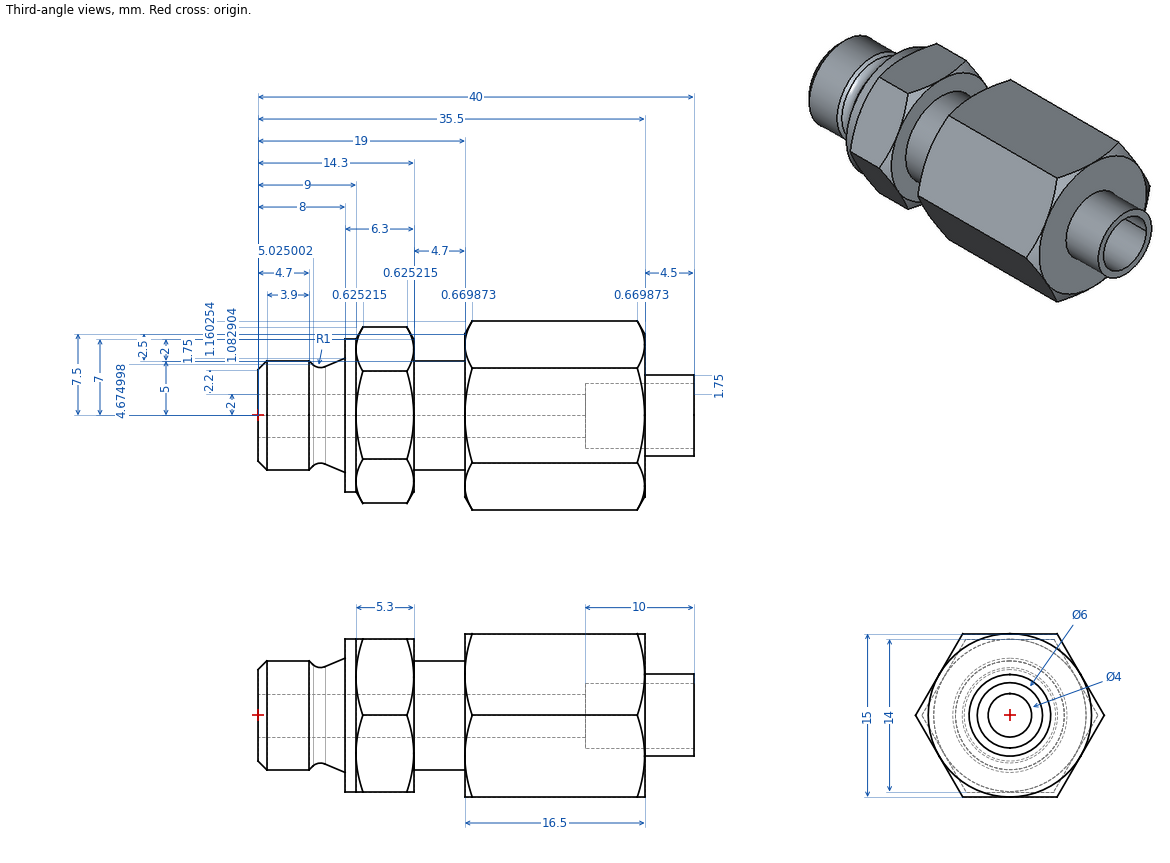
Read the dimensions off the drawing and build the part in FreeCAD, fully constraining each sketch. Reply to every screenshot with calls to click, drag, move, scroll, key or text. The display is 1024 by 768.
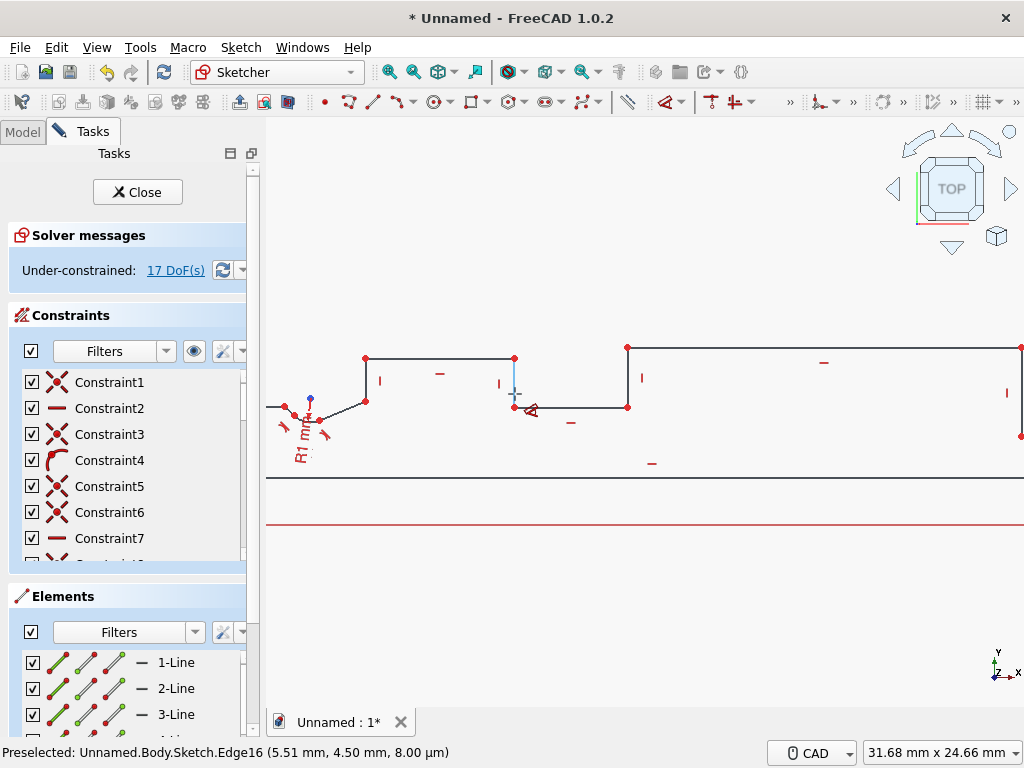
click(514, 393)
click(480, 383)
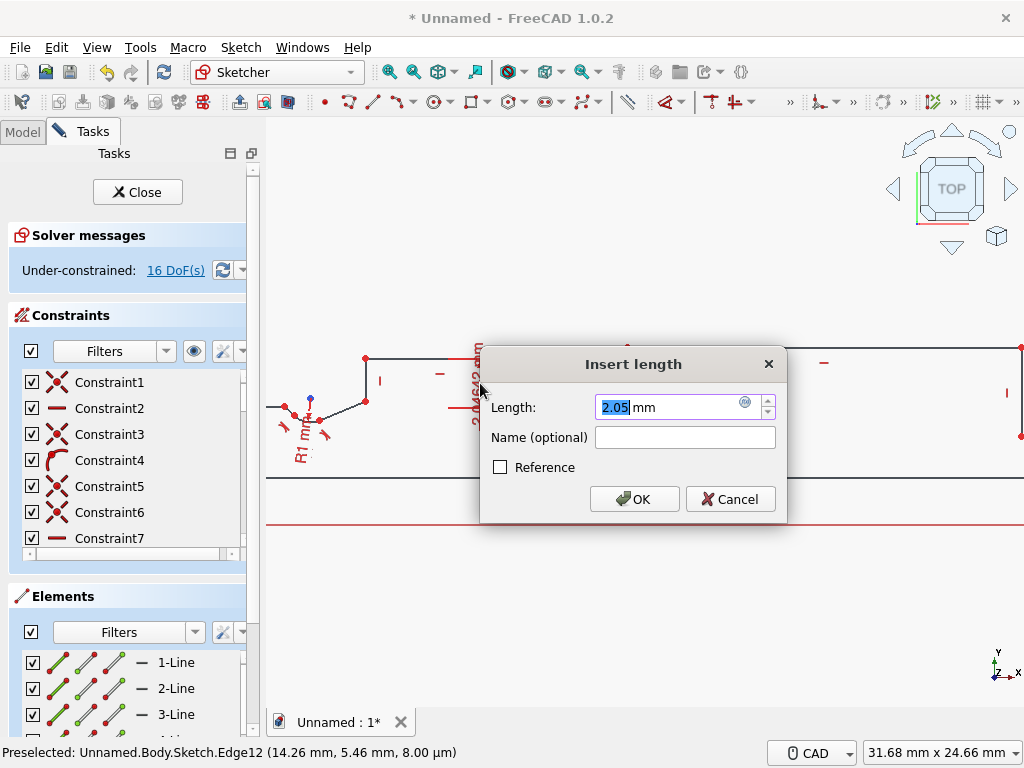
text(2)
key(Return)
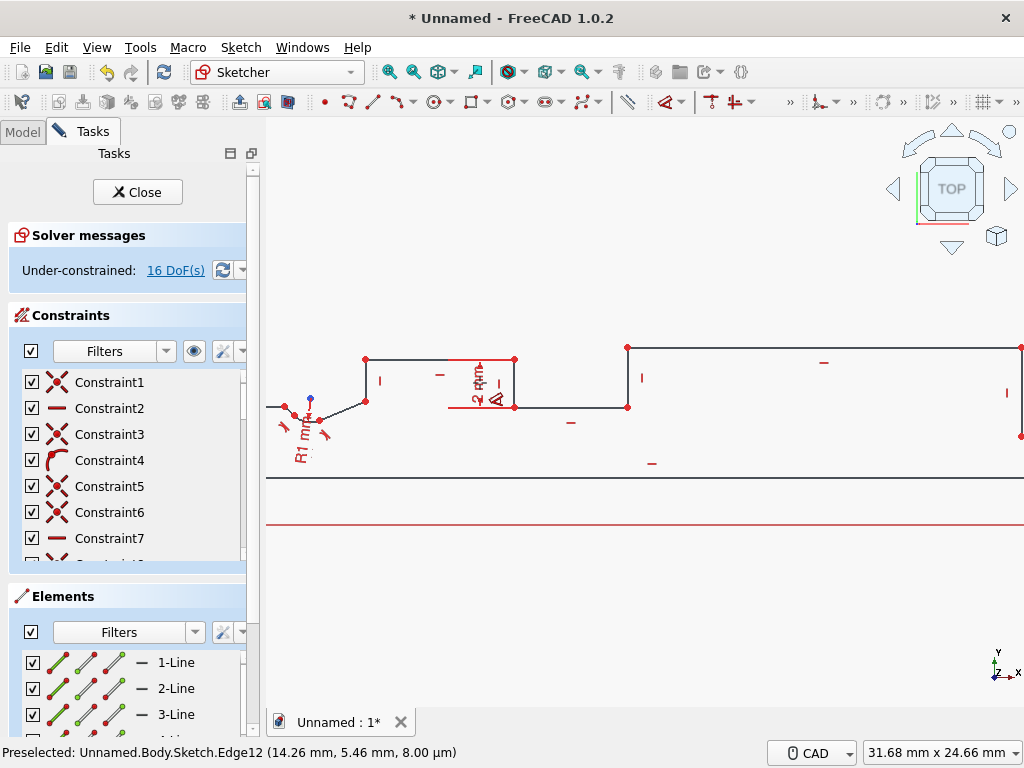
click(461, 478)
click(576, 444)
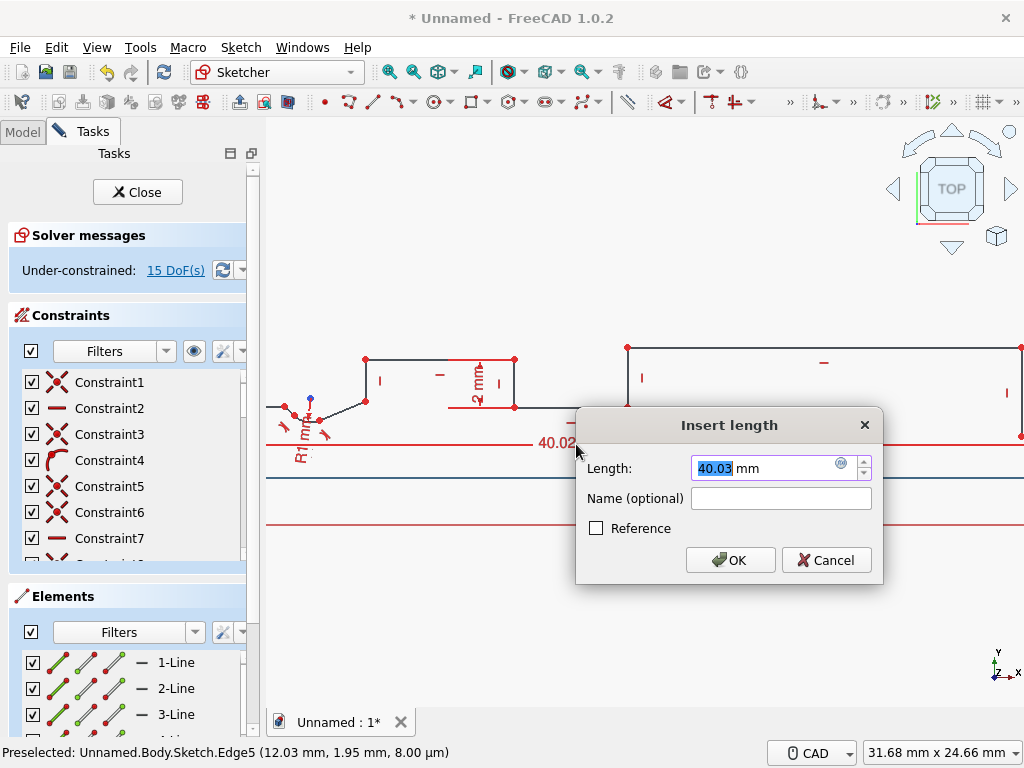
text(40)
key(Return)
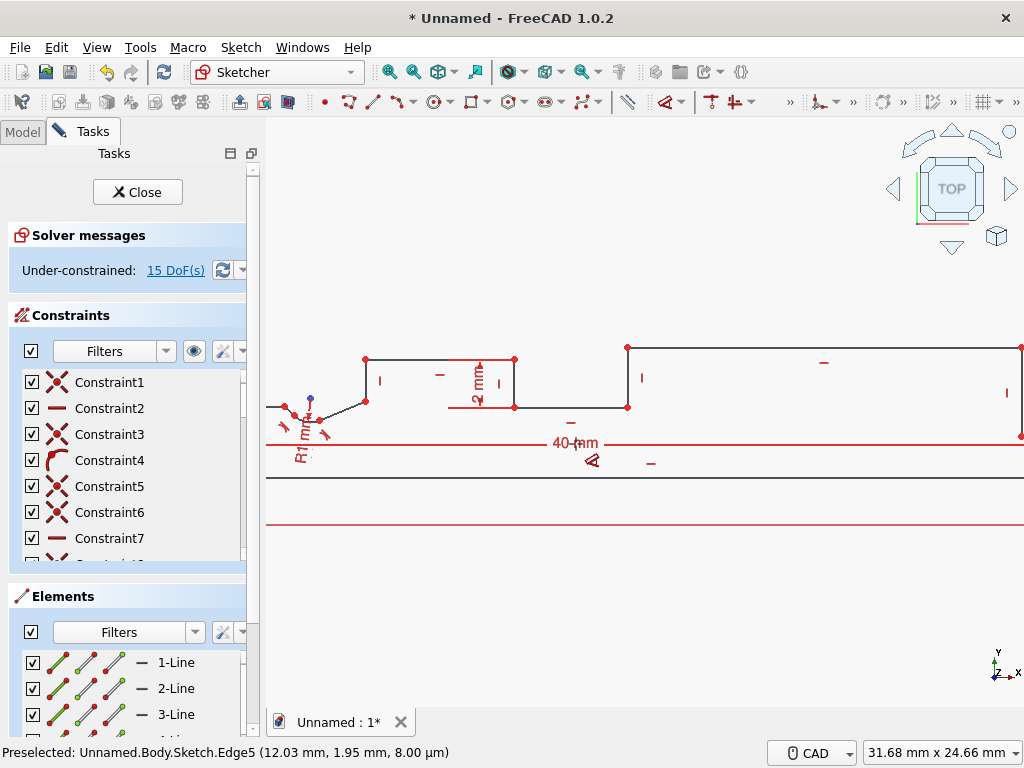
scroll(515, 393, down, 4)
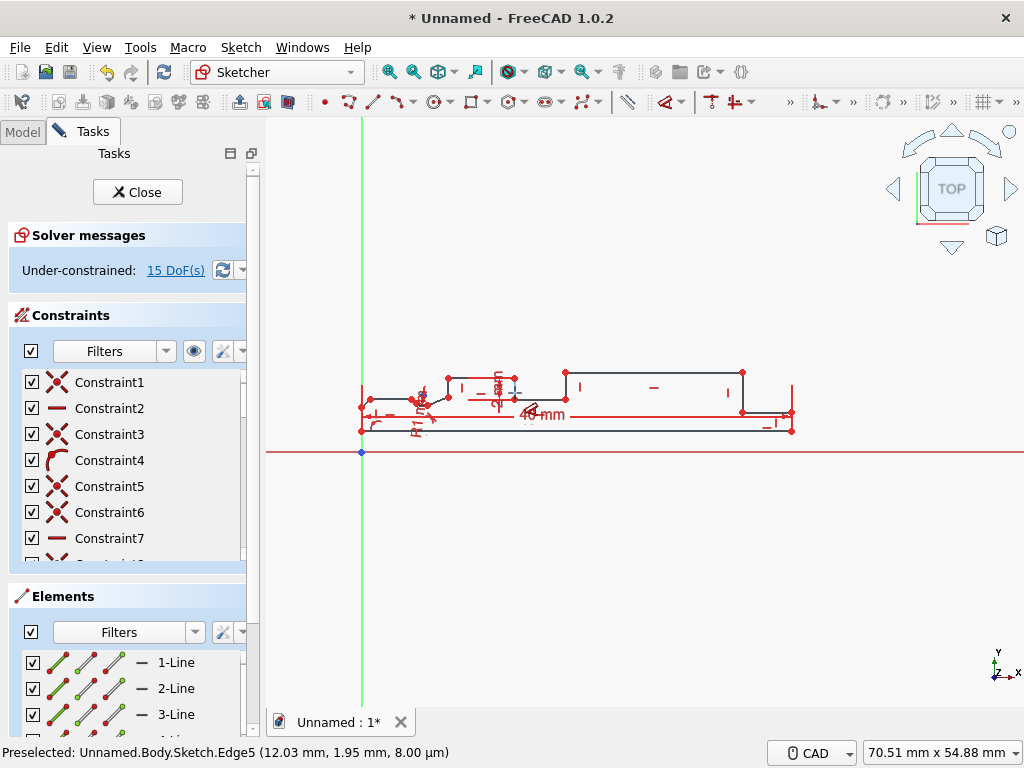
scroll(412, 399, up, 4)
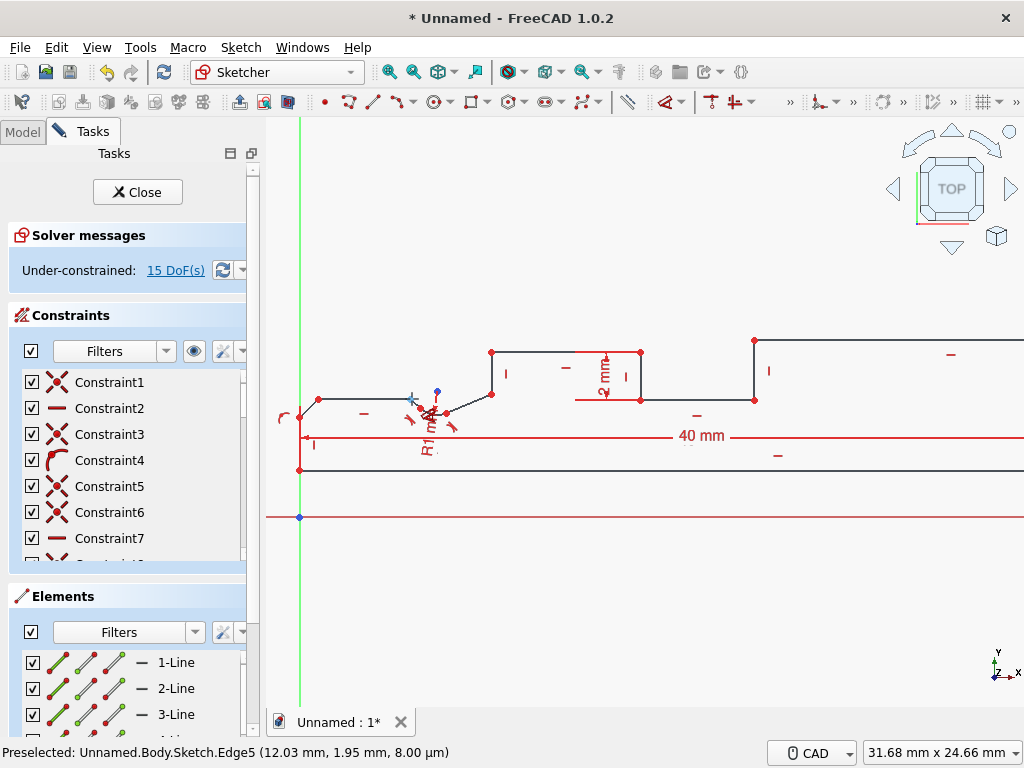
click(411, 399)
click(445, 485)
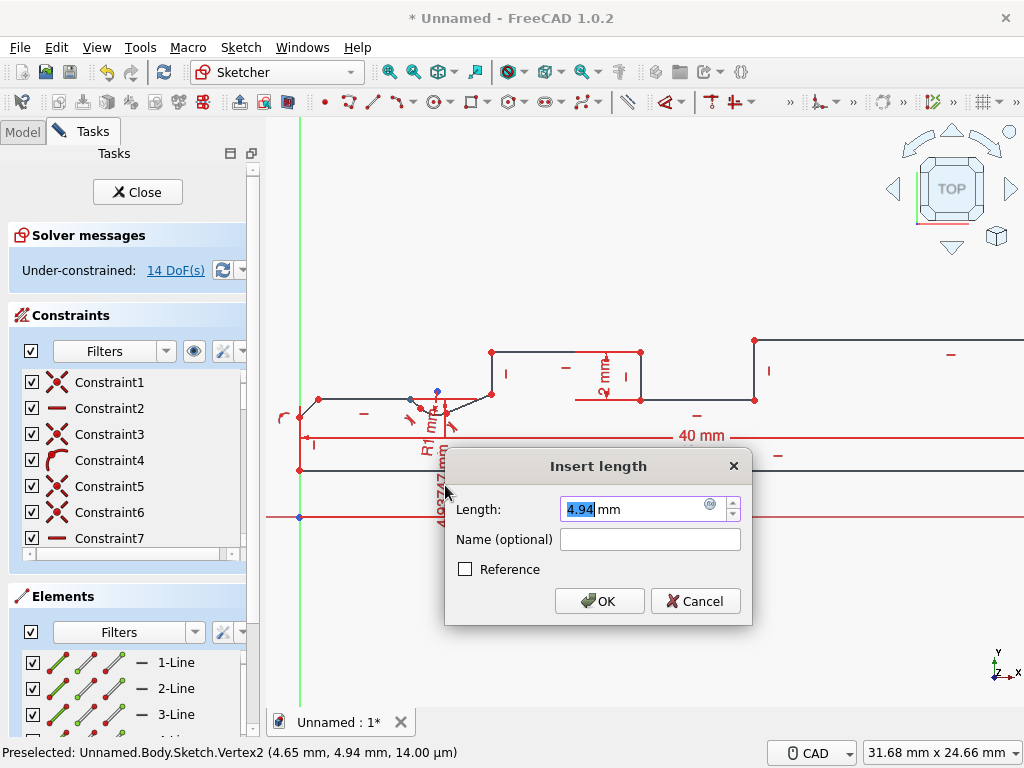
text(5)
key(Return)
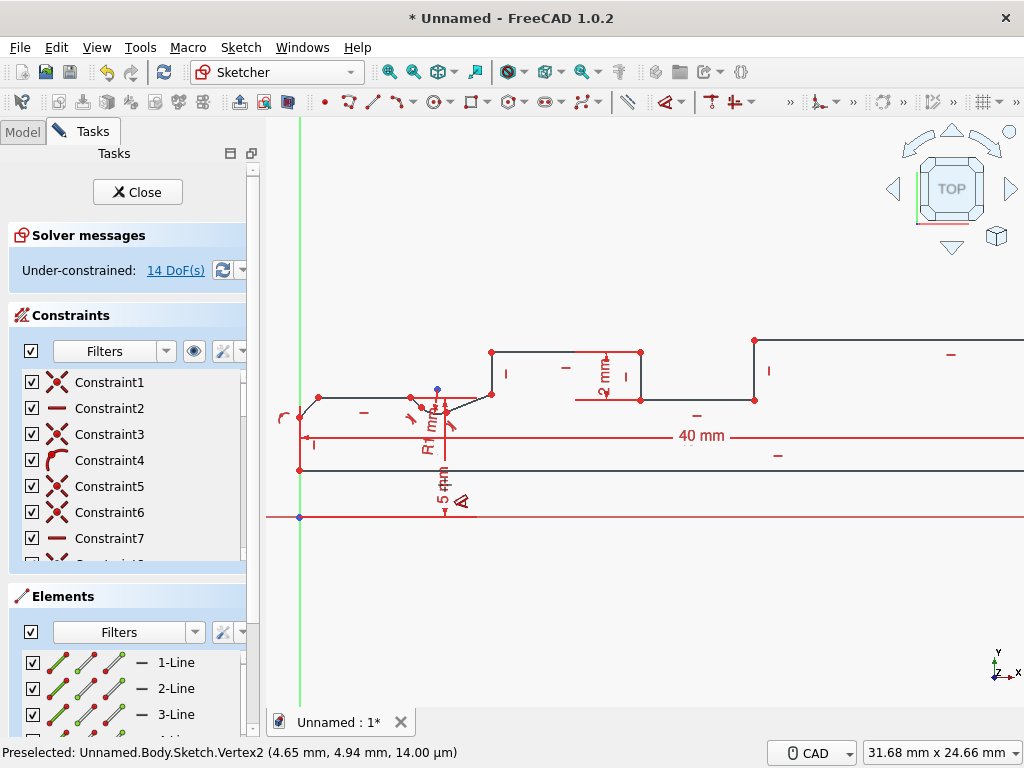
click(300, 471)
click(334, 494)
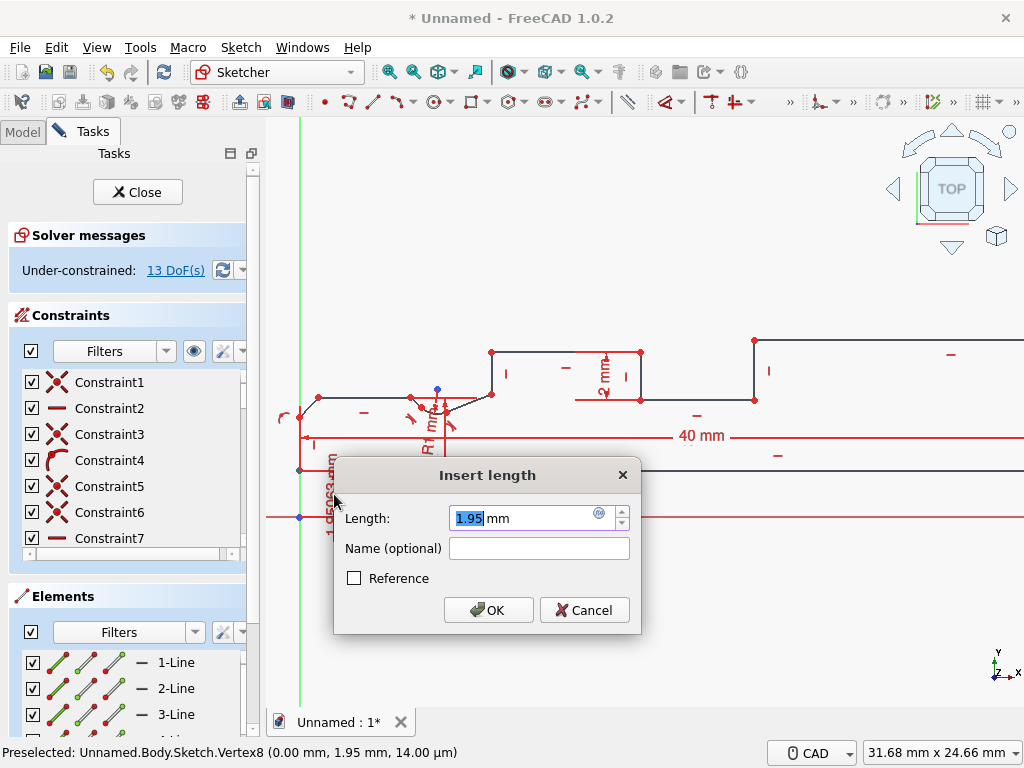
text(2)
key(Return)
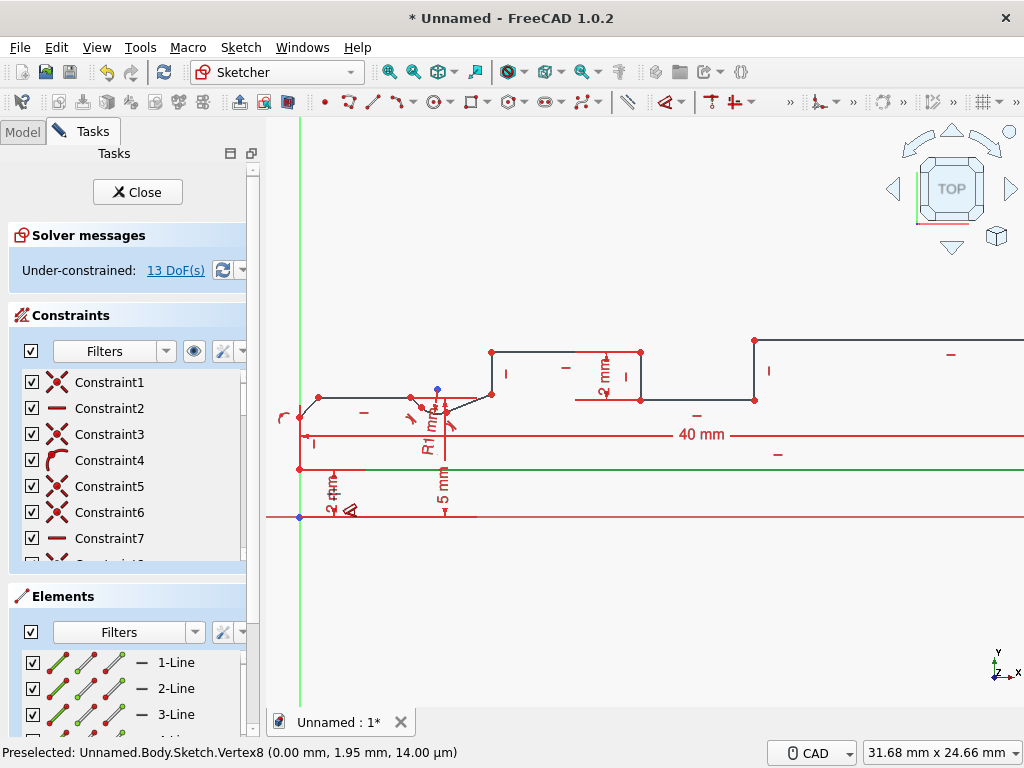
click(754, 400)
click(788, 432)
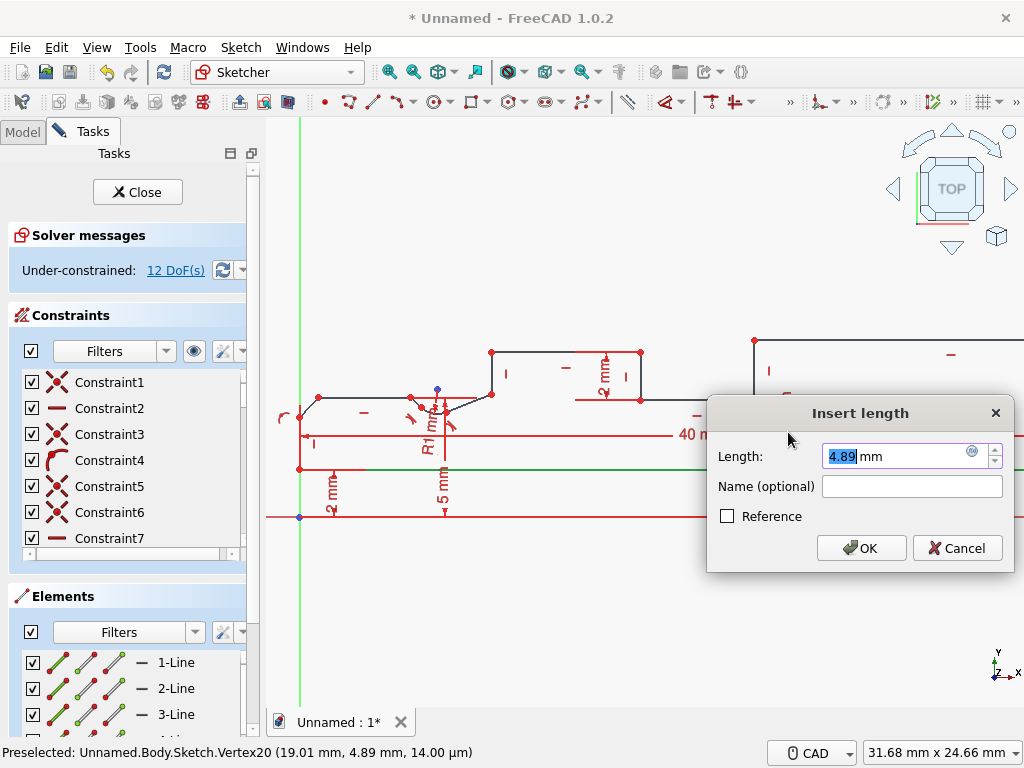
text(5)
key(Return)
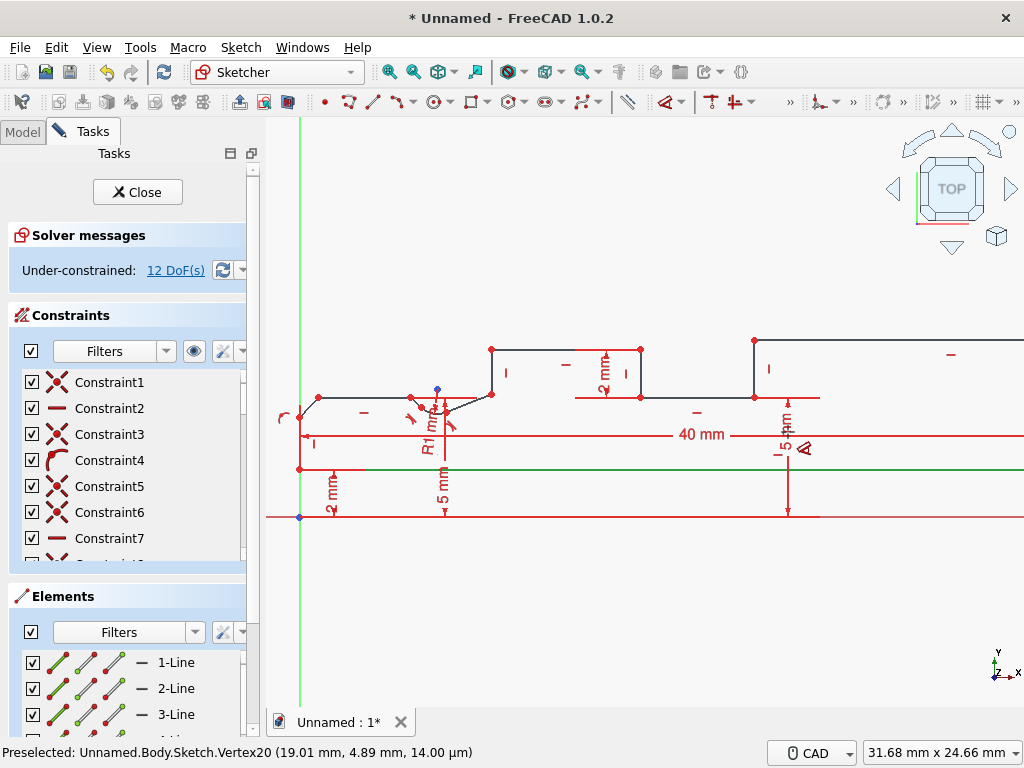
click(492, 350)
click(396, 551)